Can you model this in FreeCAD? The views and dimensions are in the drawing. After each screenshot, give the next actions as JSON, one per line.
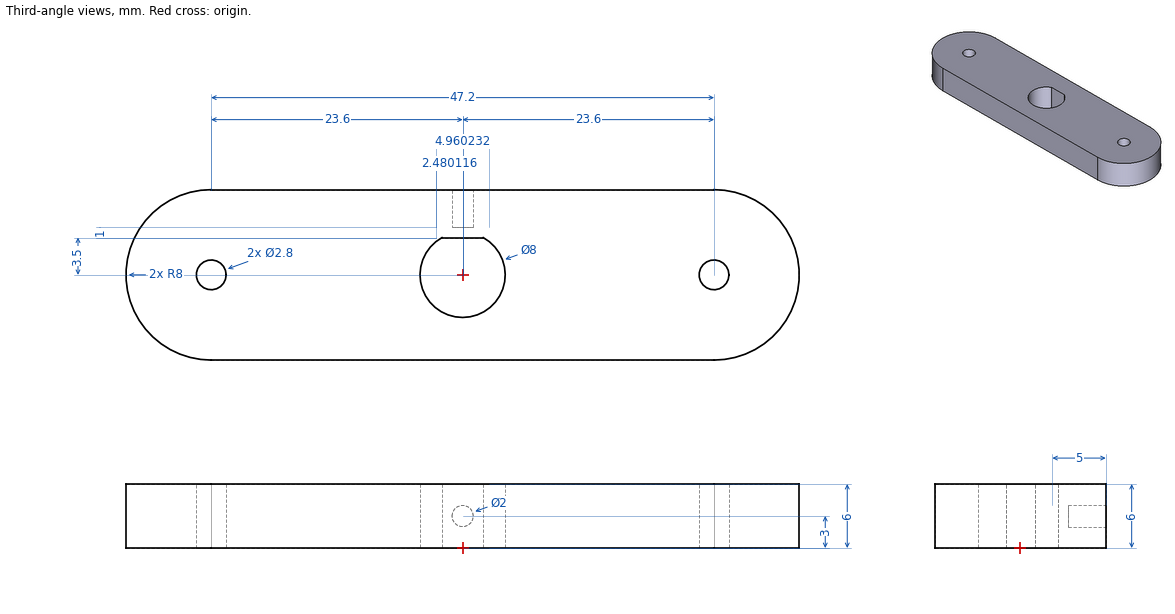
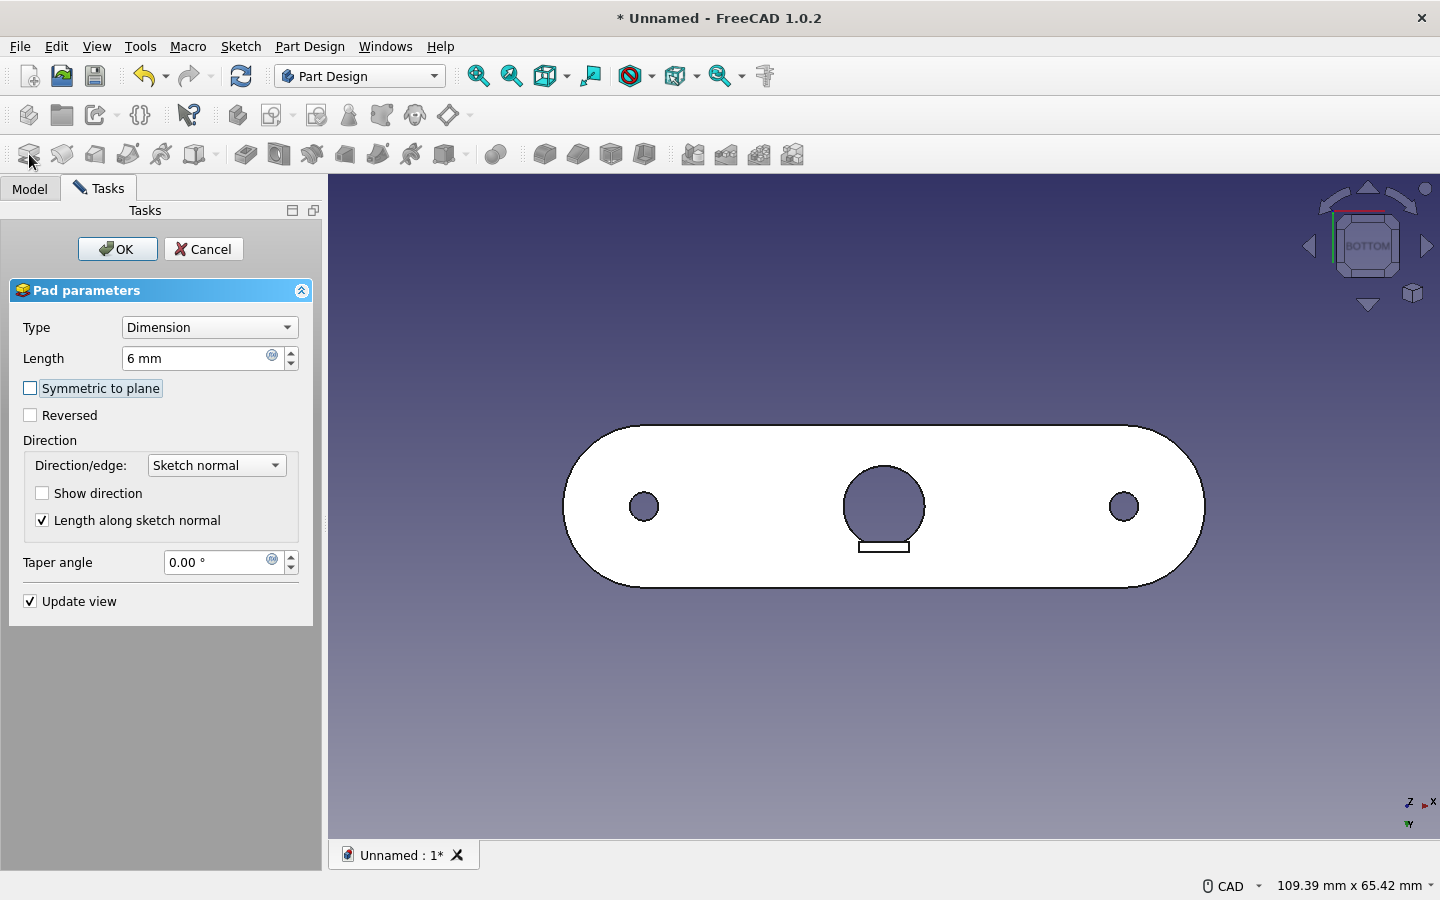
{"action": "left_click", "coordinate": [31, 415]}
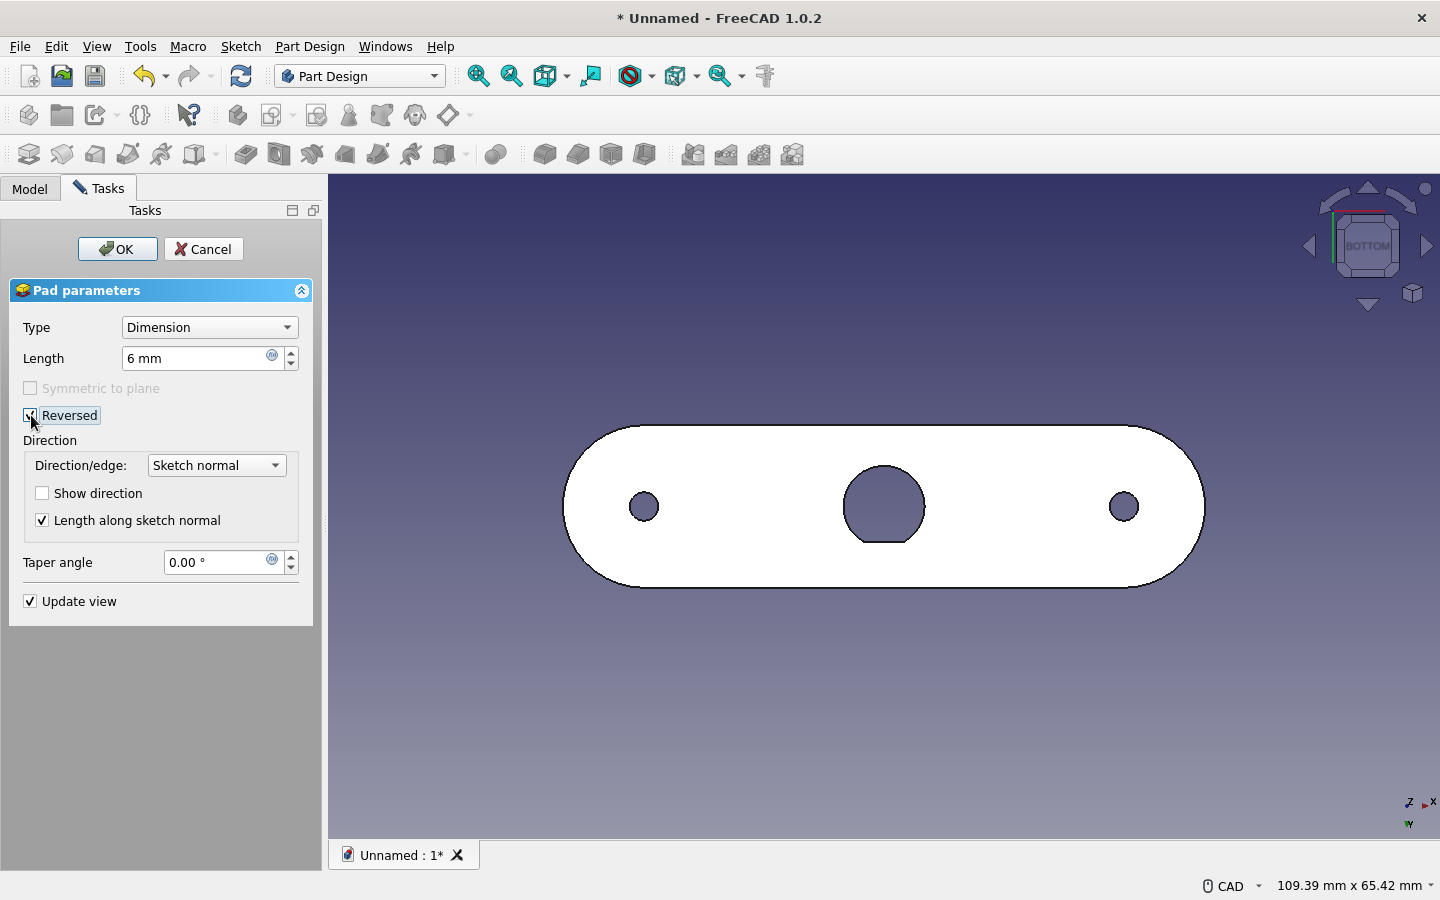
{"action": "left_click", "coordinate": [118, 249]}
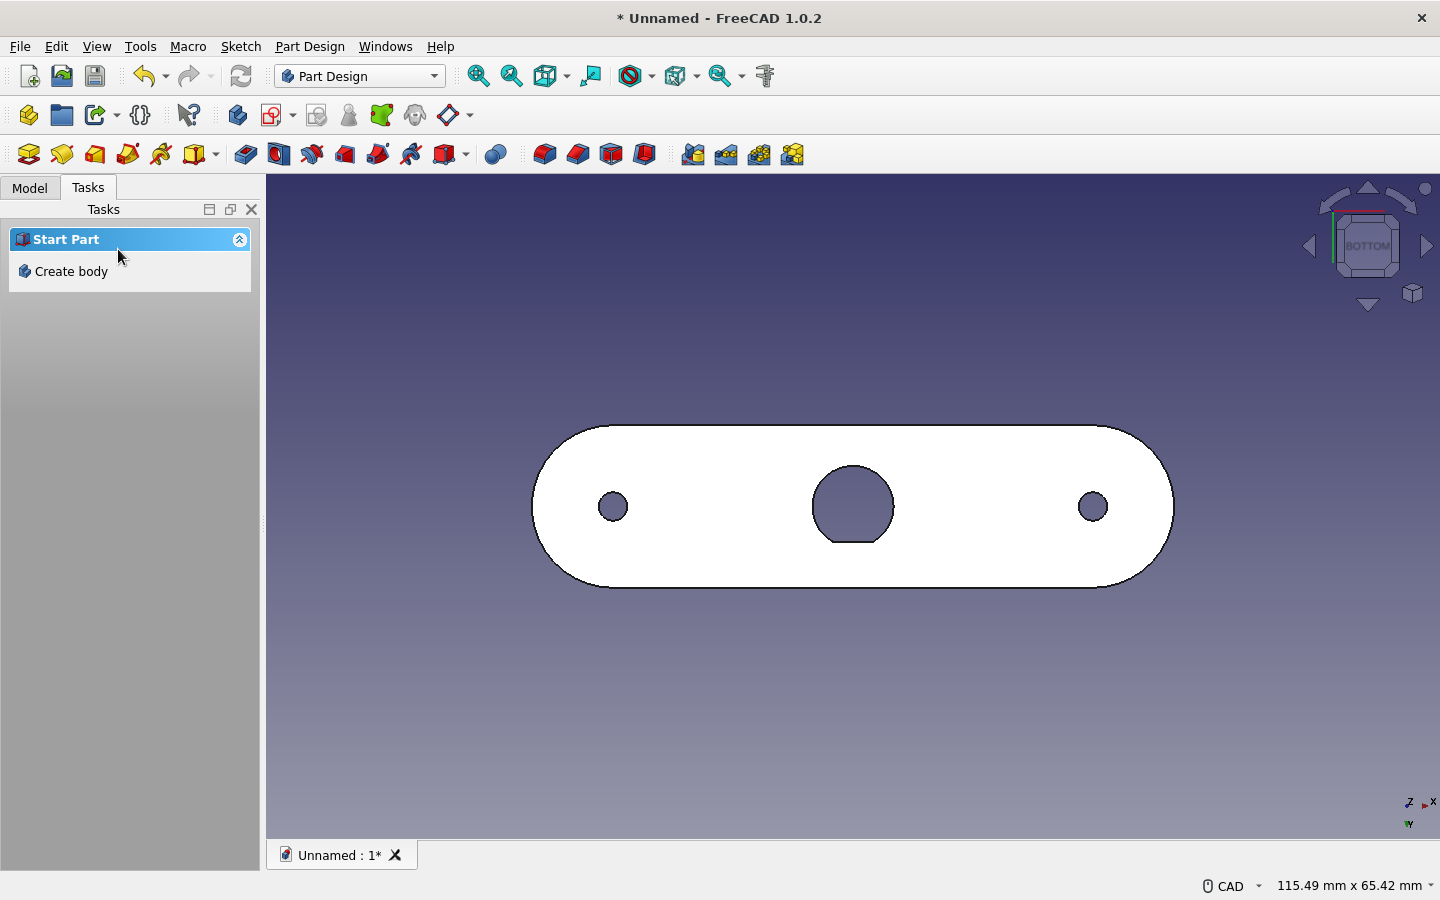
{"action": "key", "text": "0"}